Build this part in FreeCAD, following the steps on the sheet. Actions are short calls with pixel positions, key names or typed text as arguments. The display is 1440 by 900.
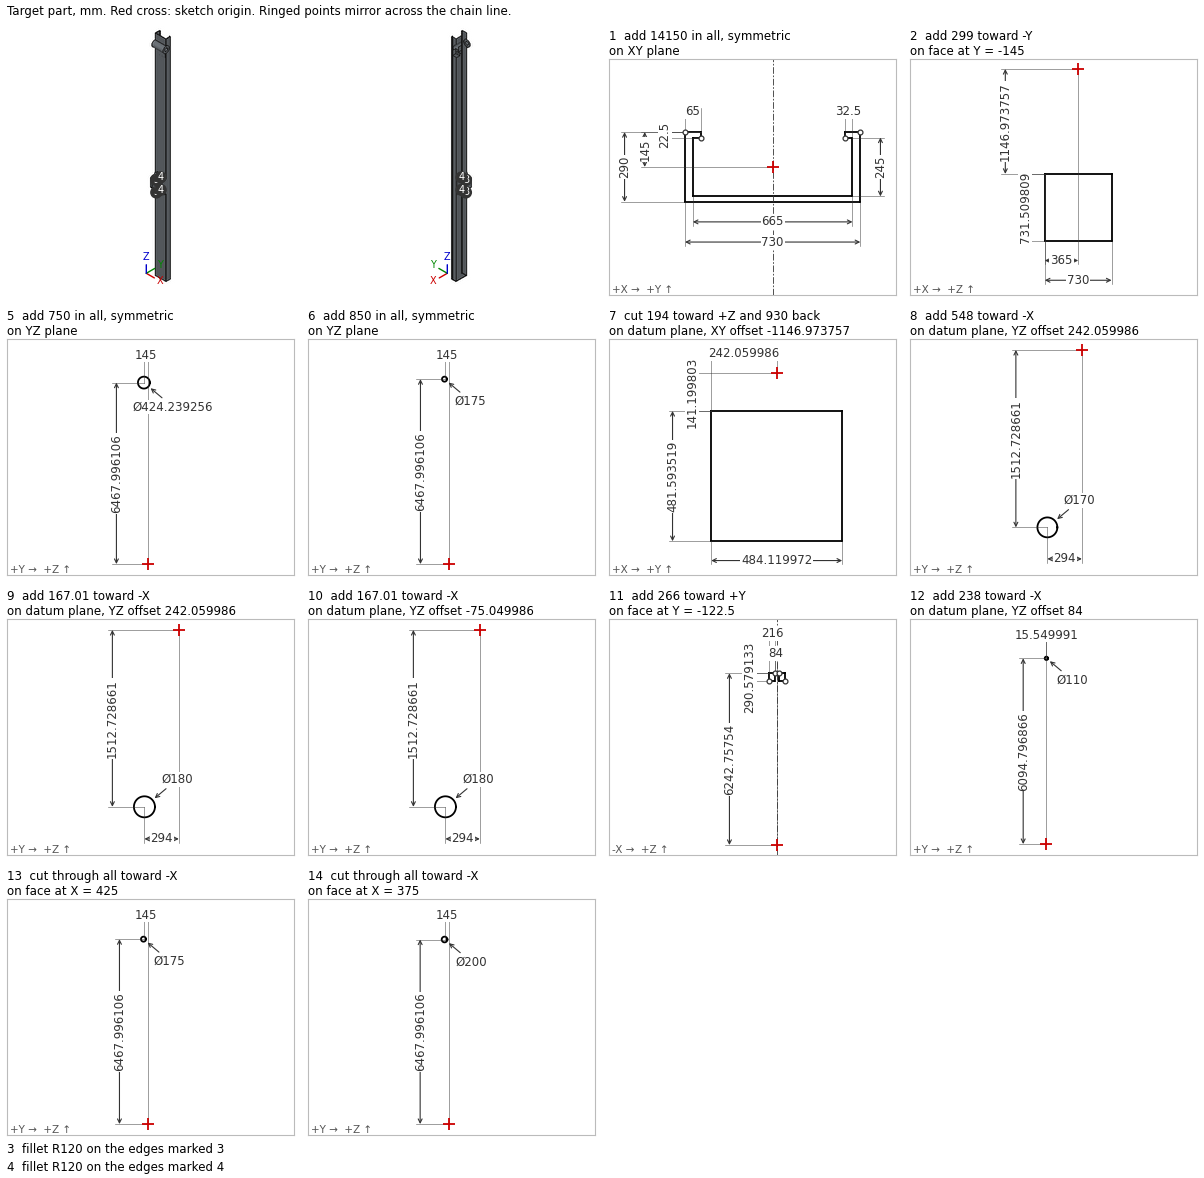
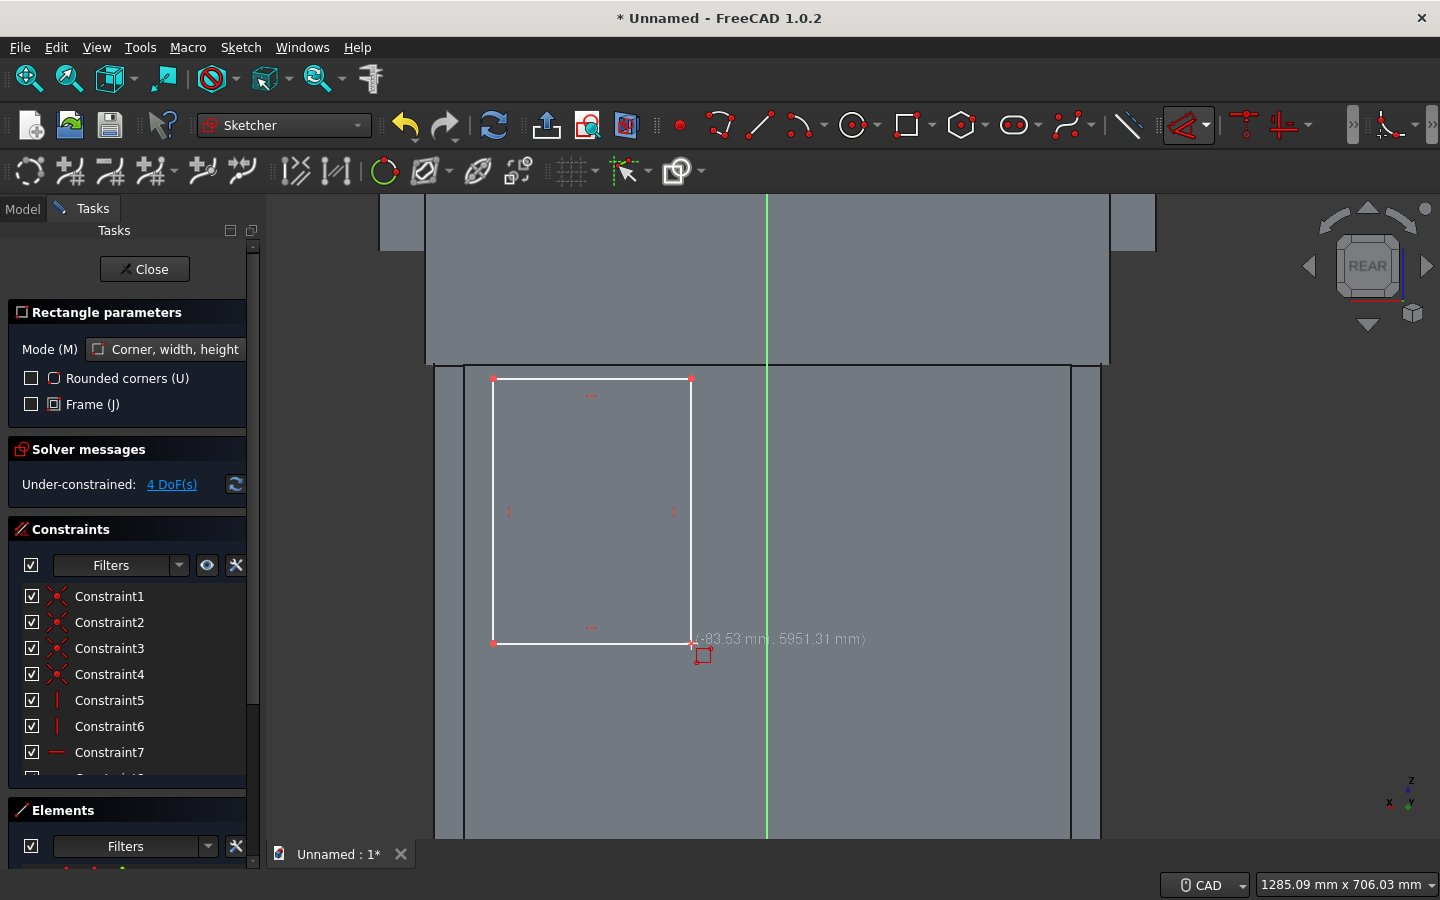
click(844, 378)
click(1041, 643)
key(Escape)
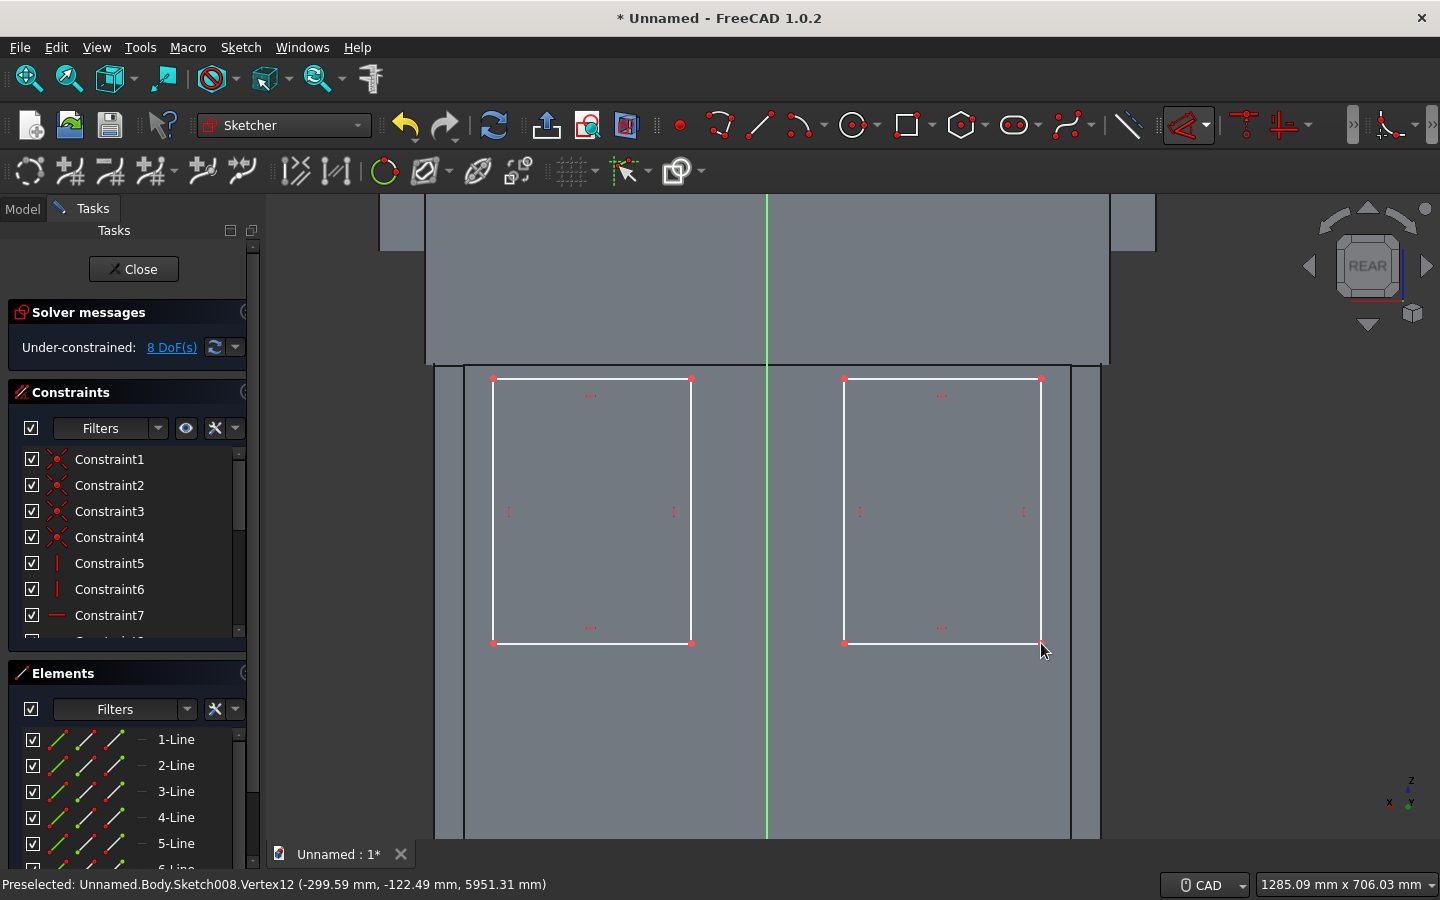
click(691, 379)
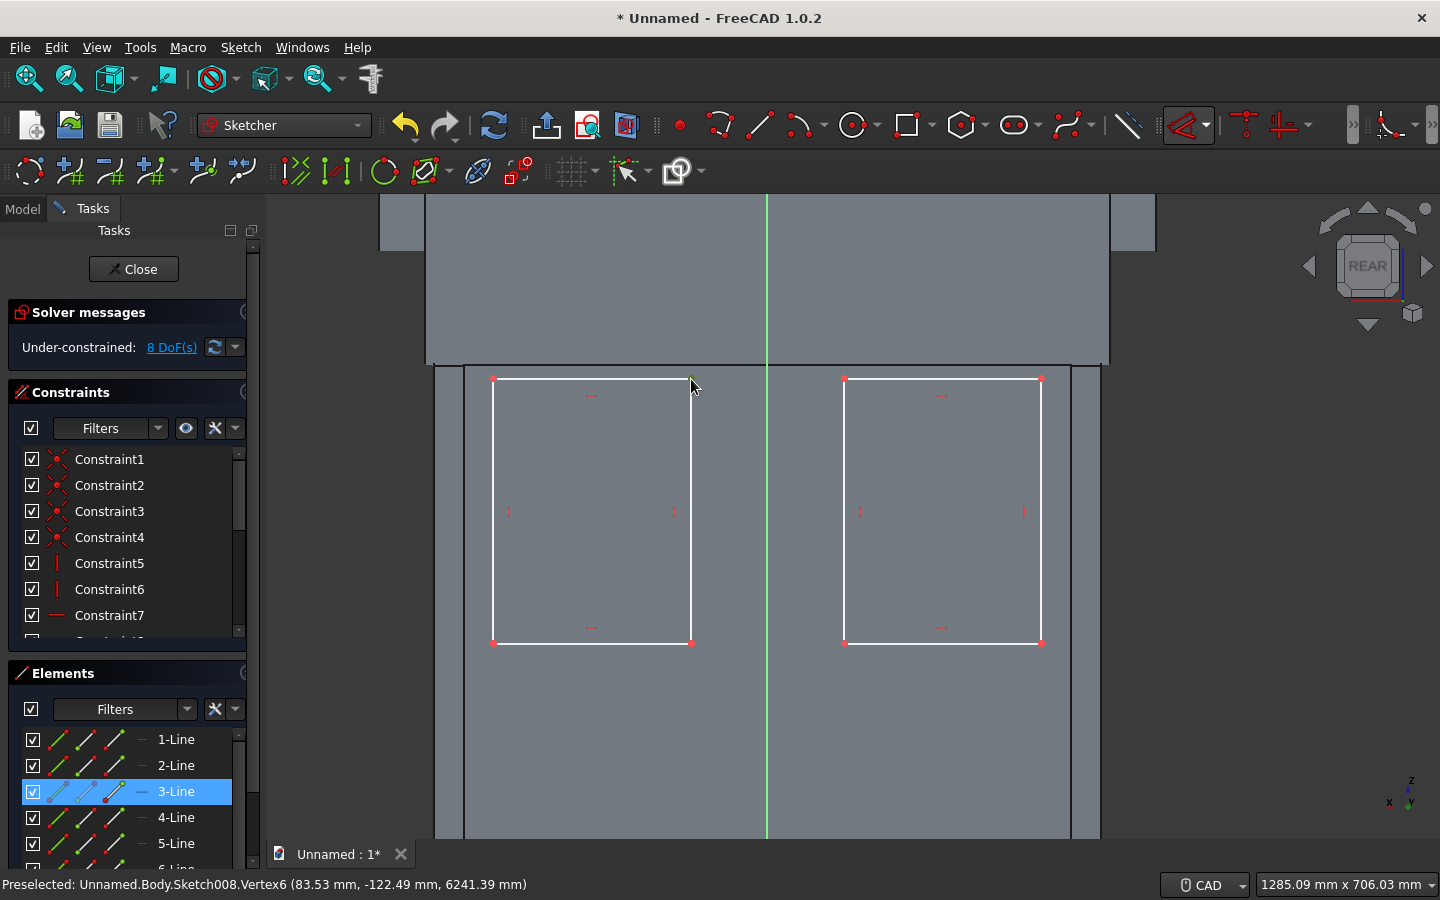
click(844, 379)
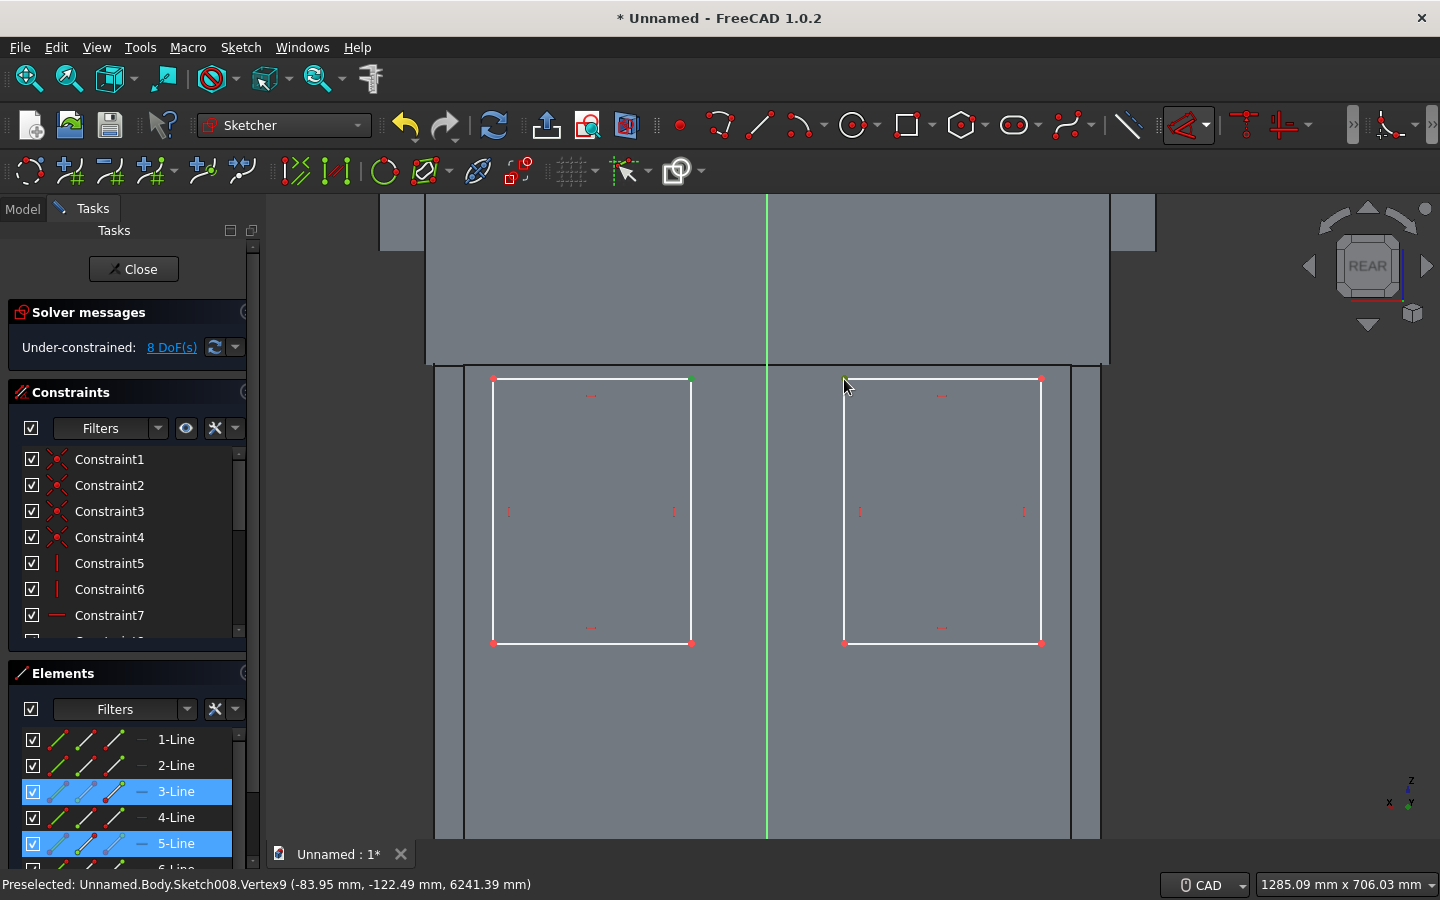
click(767, 769)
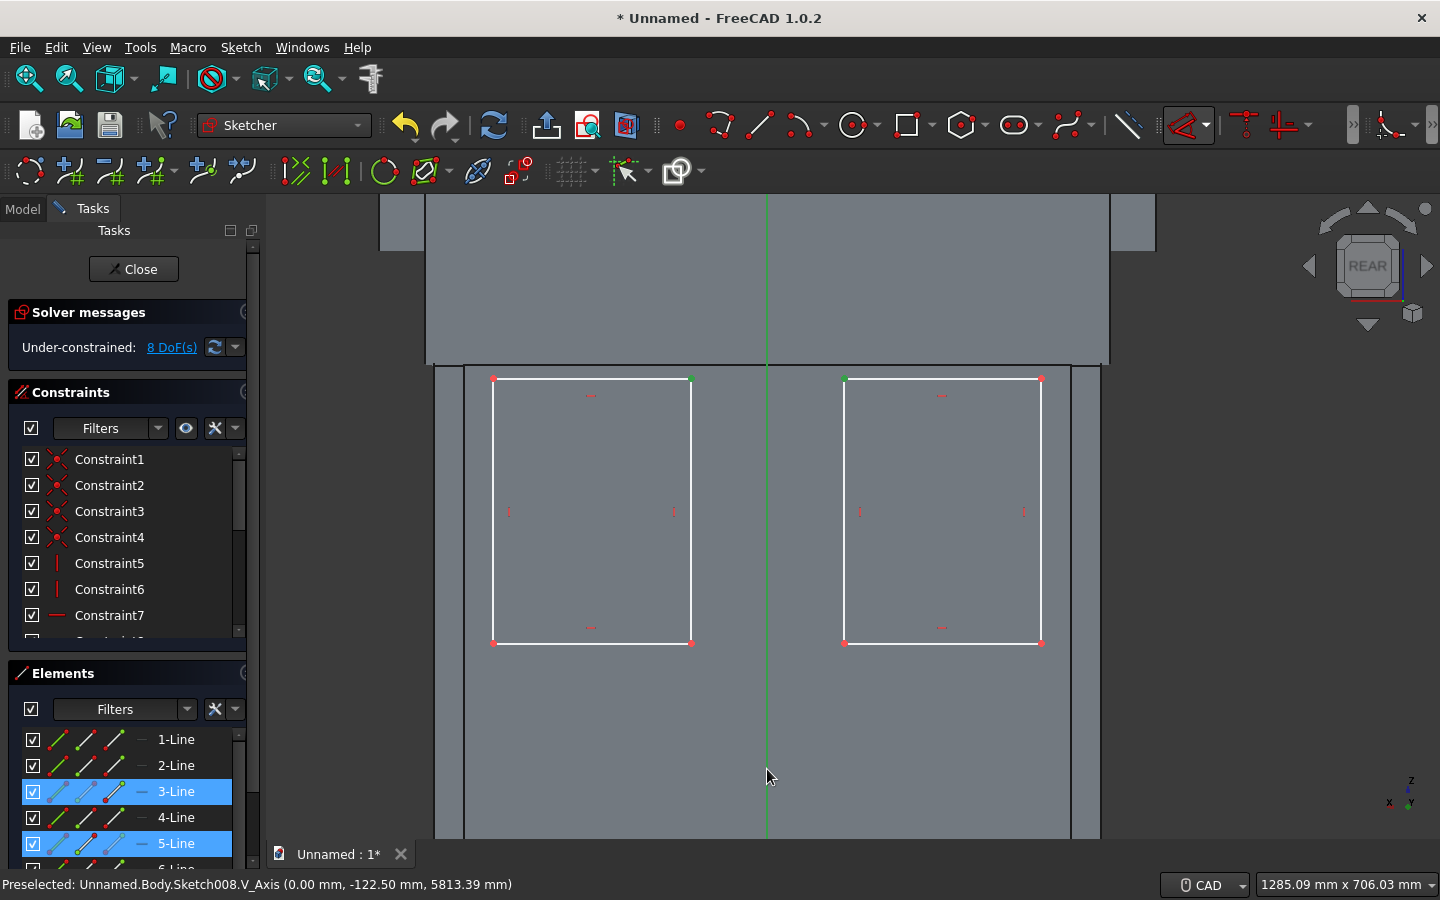
key(s)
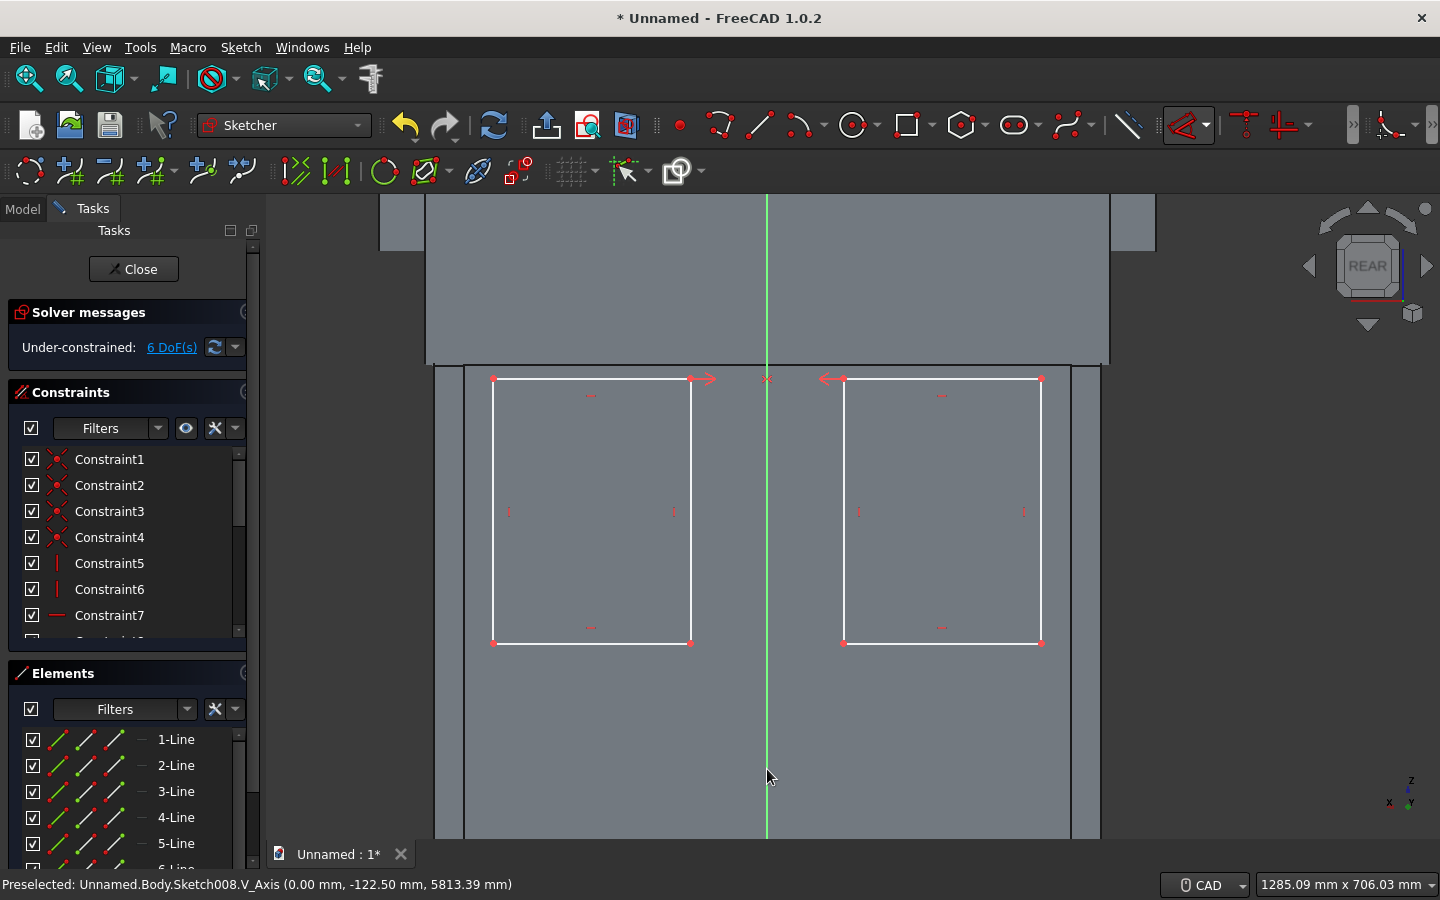
click(493, 644)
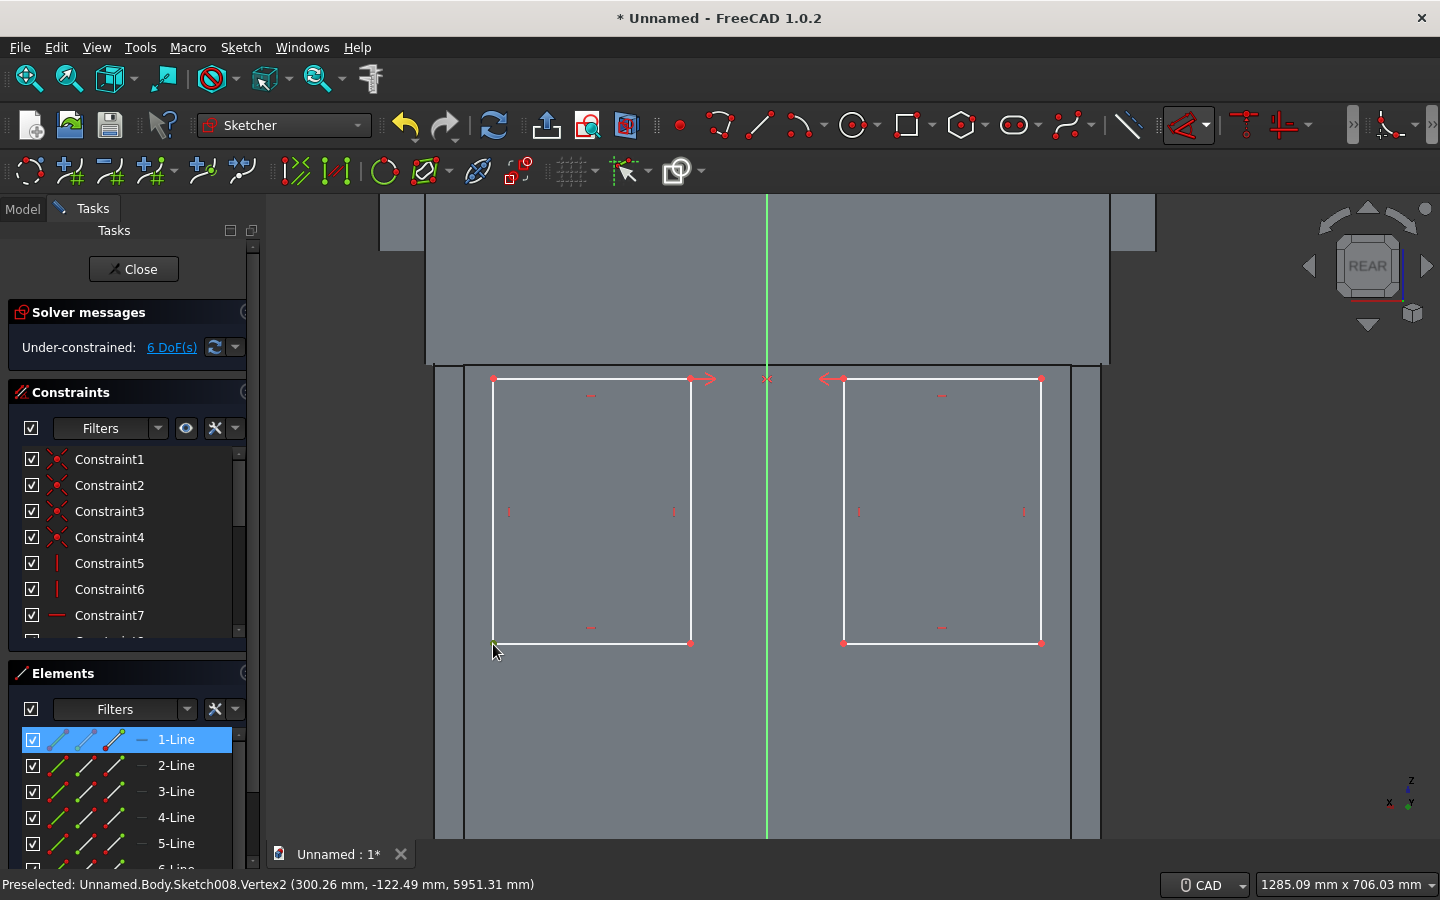
click(1041, 644)